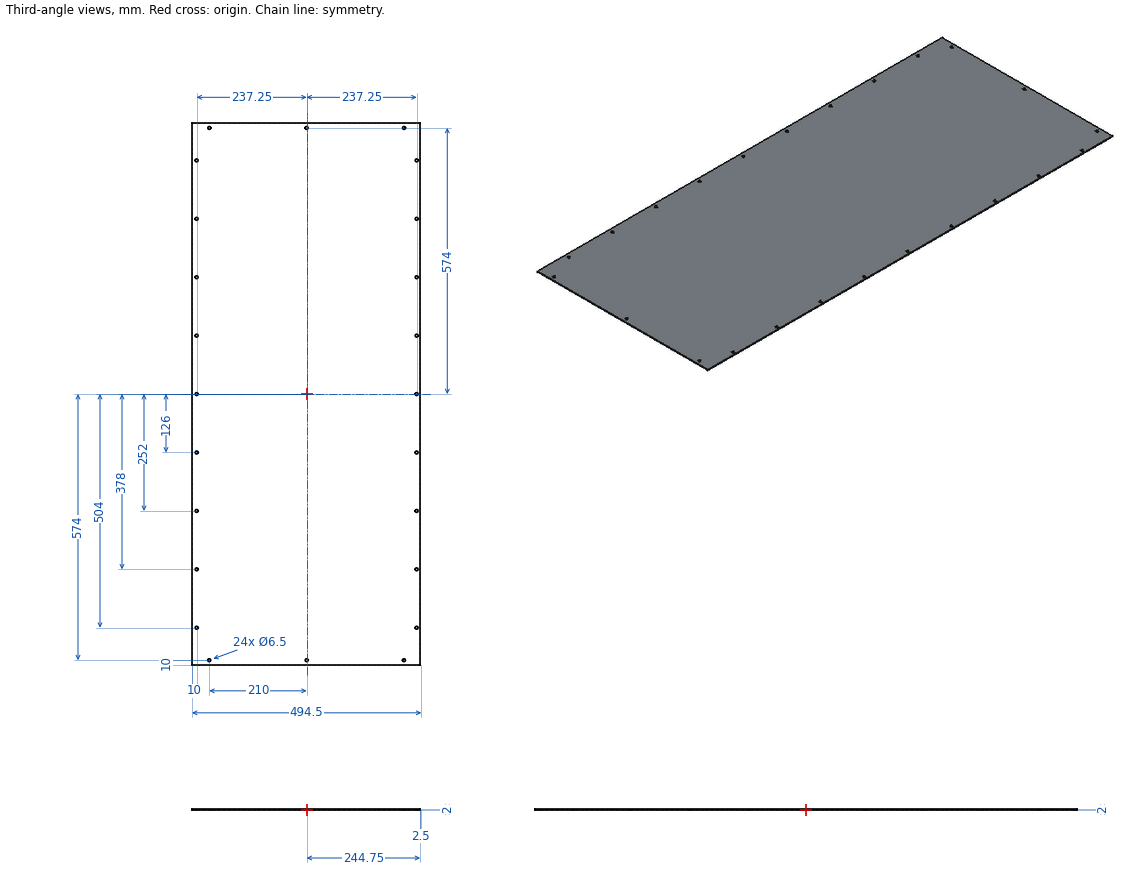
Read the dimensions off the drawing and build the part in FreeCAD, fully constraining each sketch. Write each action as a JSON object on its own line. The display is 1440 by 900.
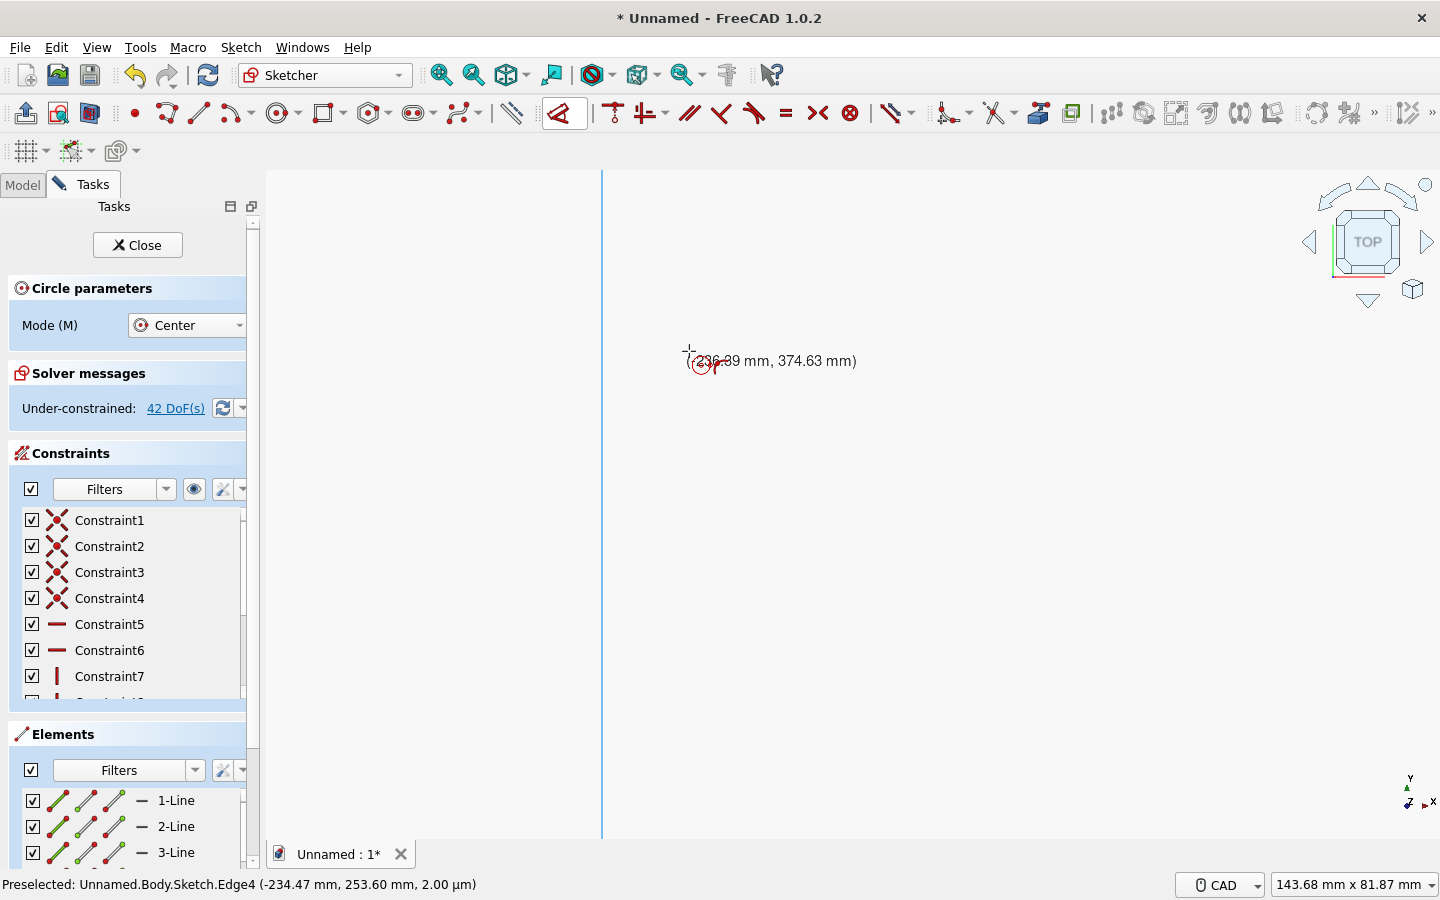
{"action": "scroll", "coordinate": [689, 351], "scroll_direction": "down", "scroll_amount": 15}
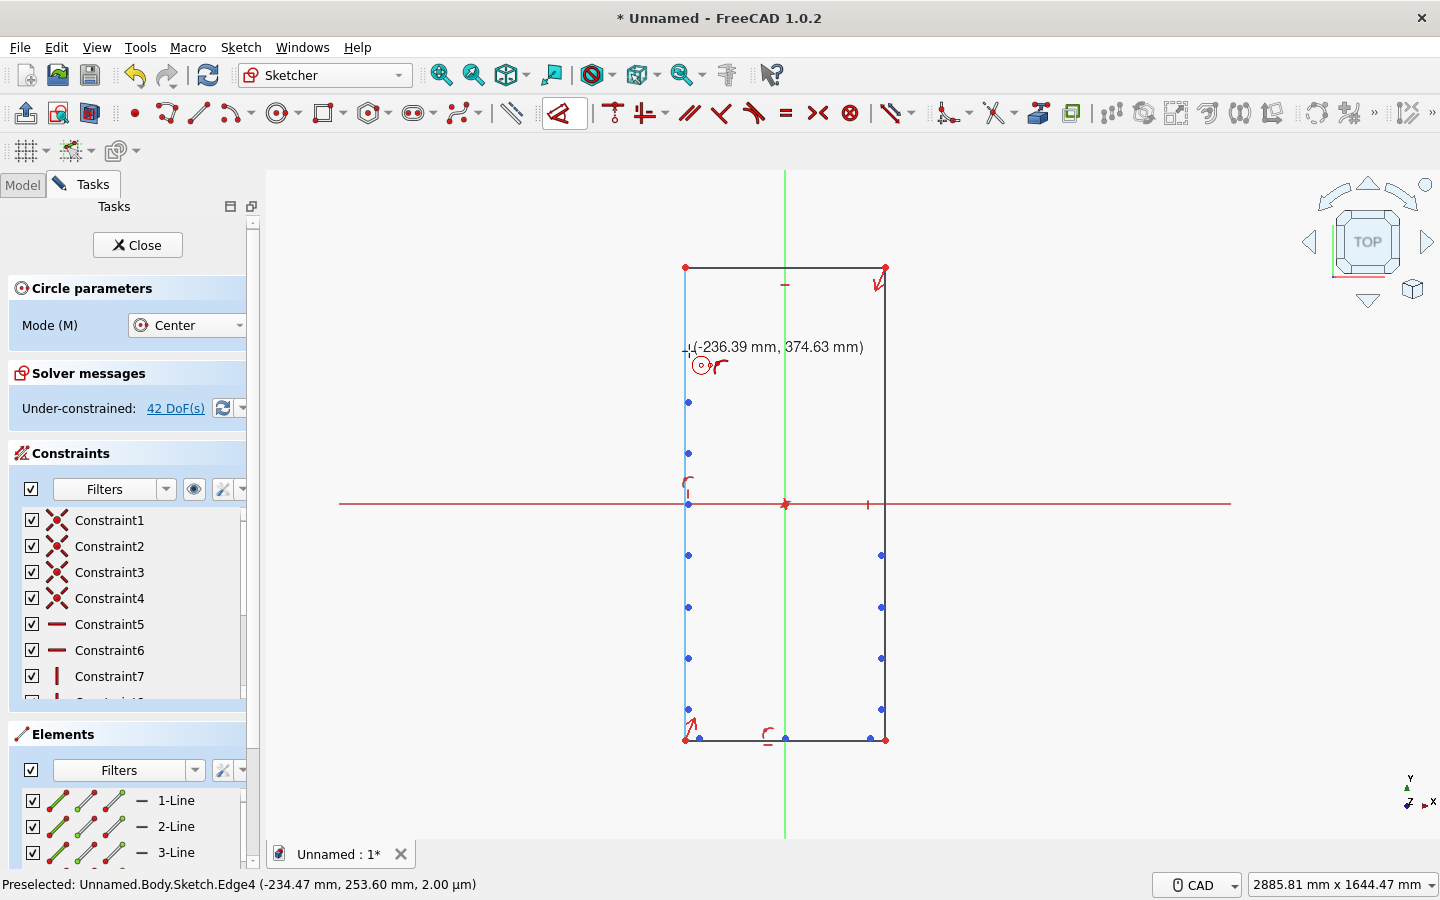
{"action": "scroll", "coordinate": [689, 351], "scroll_direction": "up", "scroll_amount": 7}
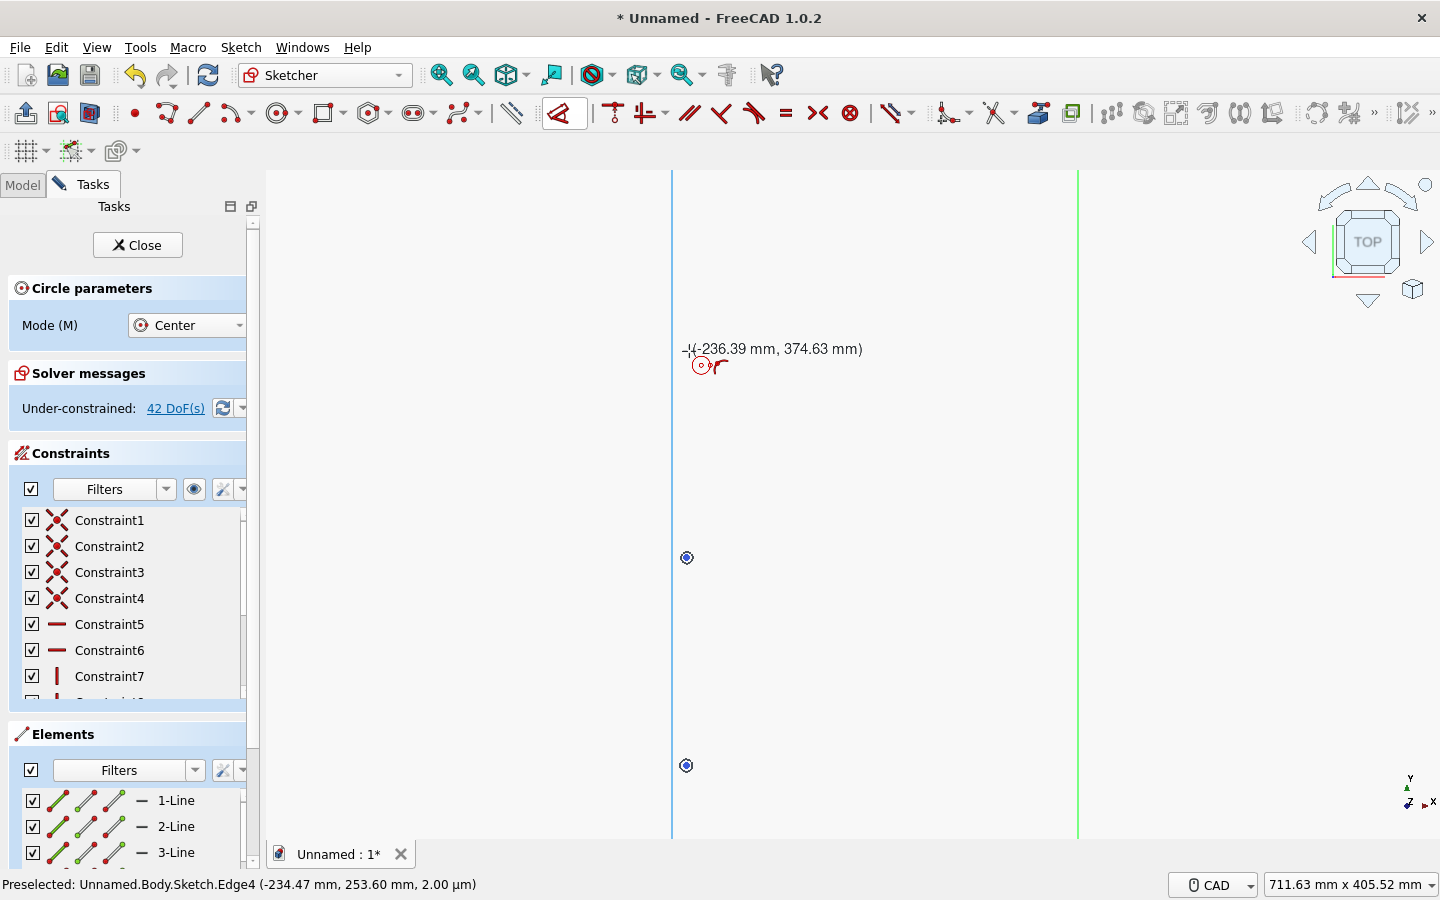
{"action": "left_click", "coordinate": [686, 349]}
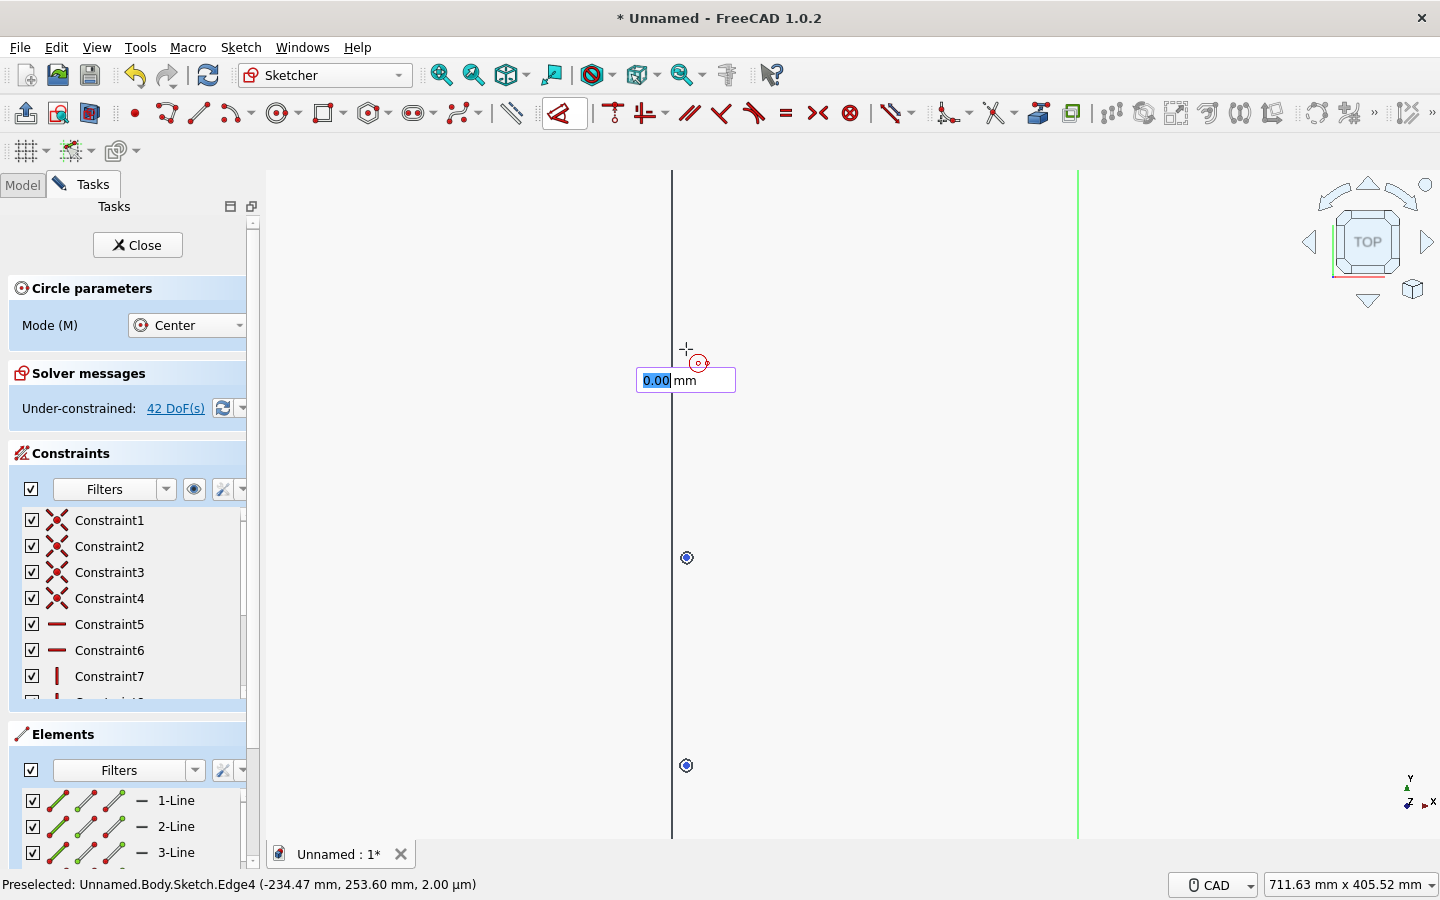
{"action": "scroll", "coordinate": [690, 345], "scroll_direction": "up", "scroll_amount": 6}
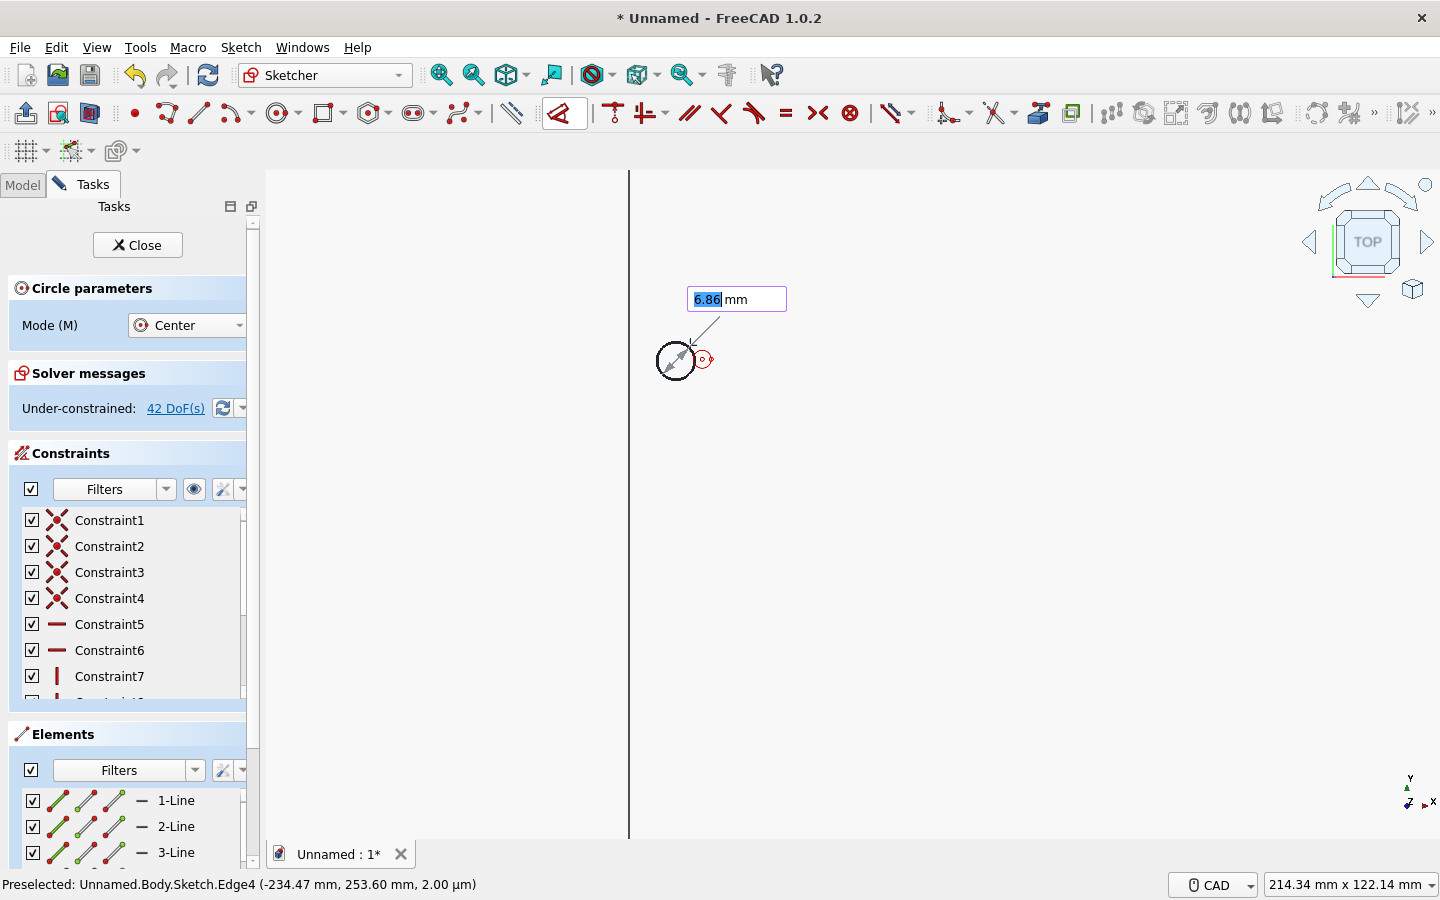
{"action": "left_click", "coordinate": [690, 344]}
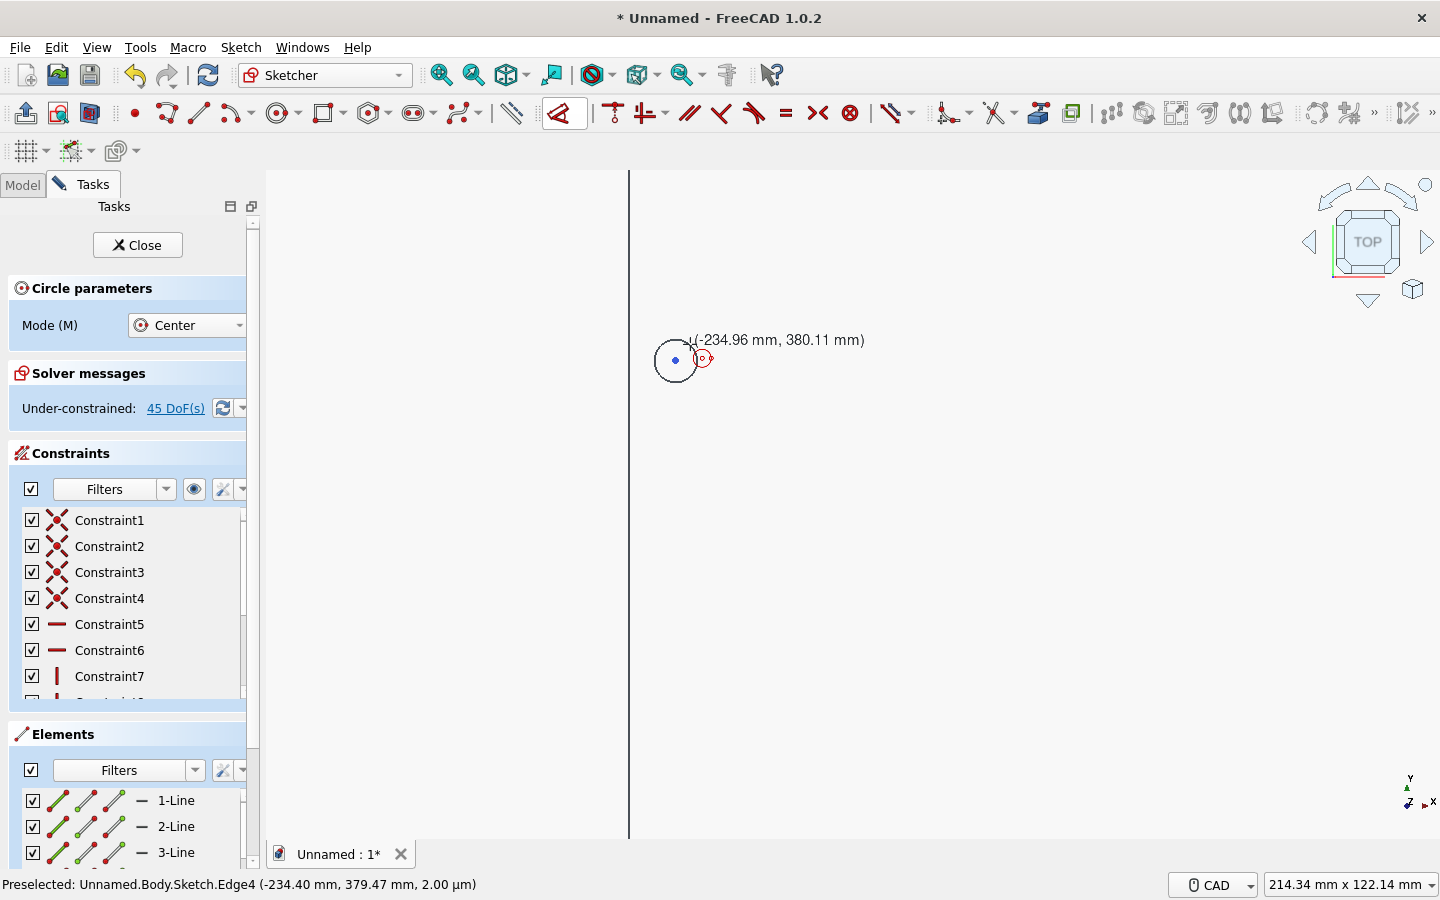
{"action": "scroll", "coordinate": [689, 350], "scroll_direction": "down", "scroll_amount": 13}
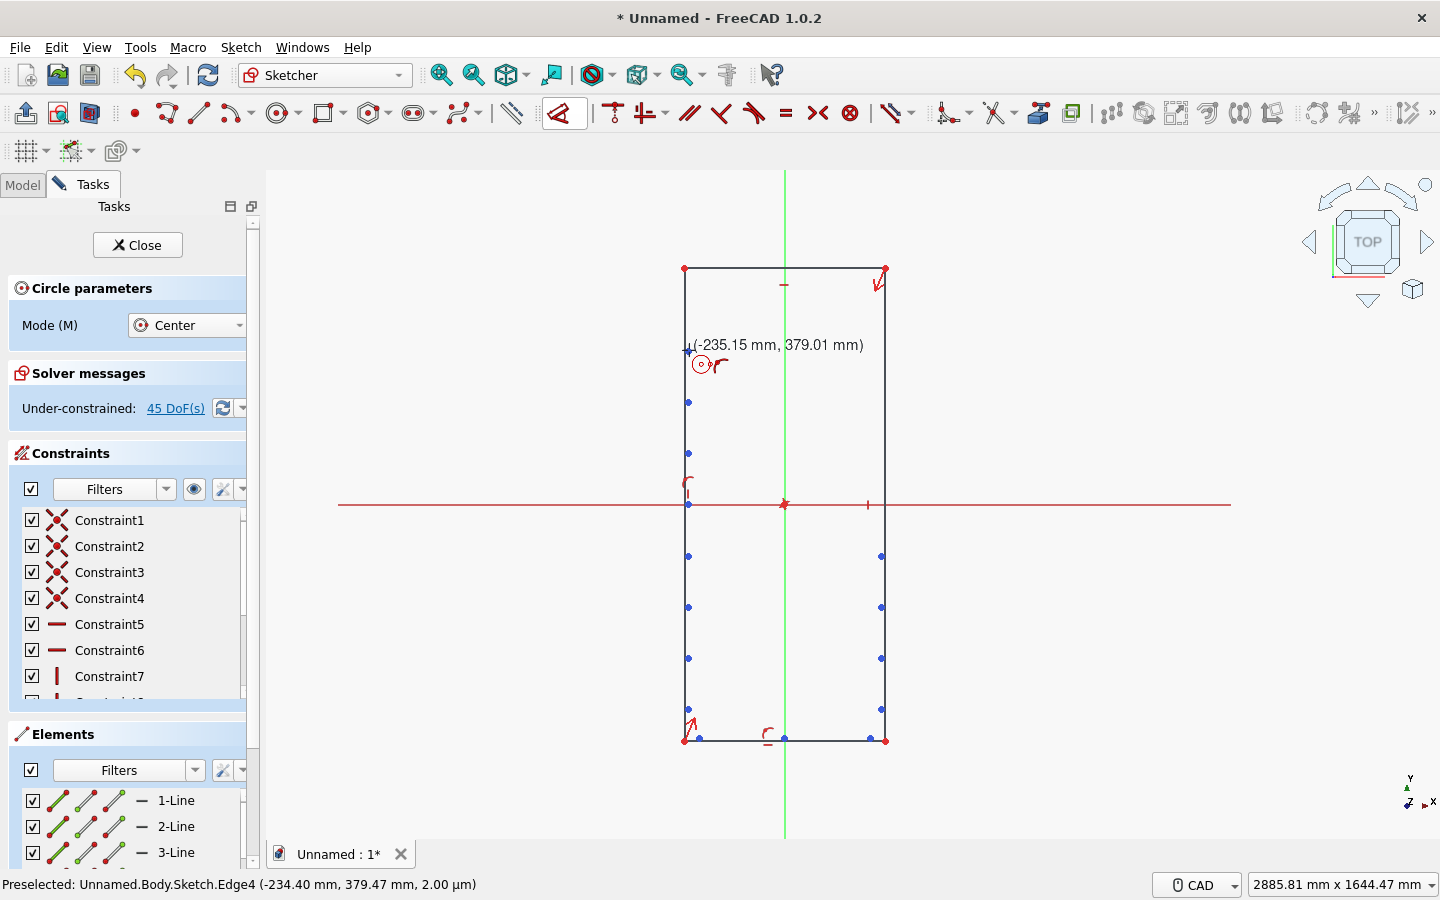
{"action": "scroll", "coordinate": [688, 299], "scroll_direction": "up", "scroll_amount": 15}